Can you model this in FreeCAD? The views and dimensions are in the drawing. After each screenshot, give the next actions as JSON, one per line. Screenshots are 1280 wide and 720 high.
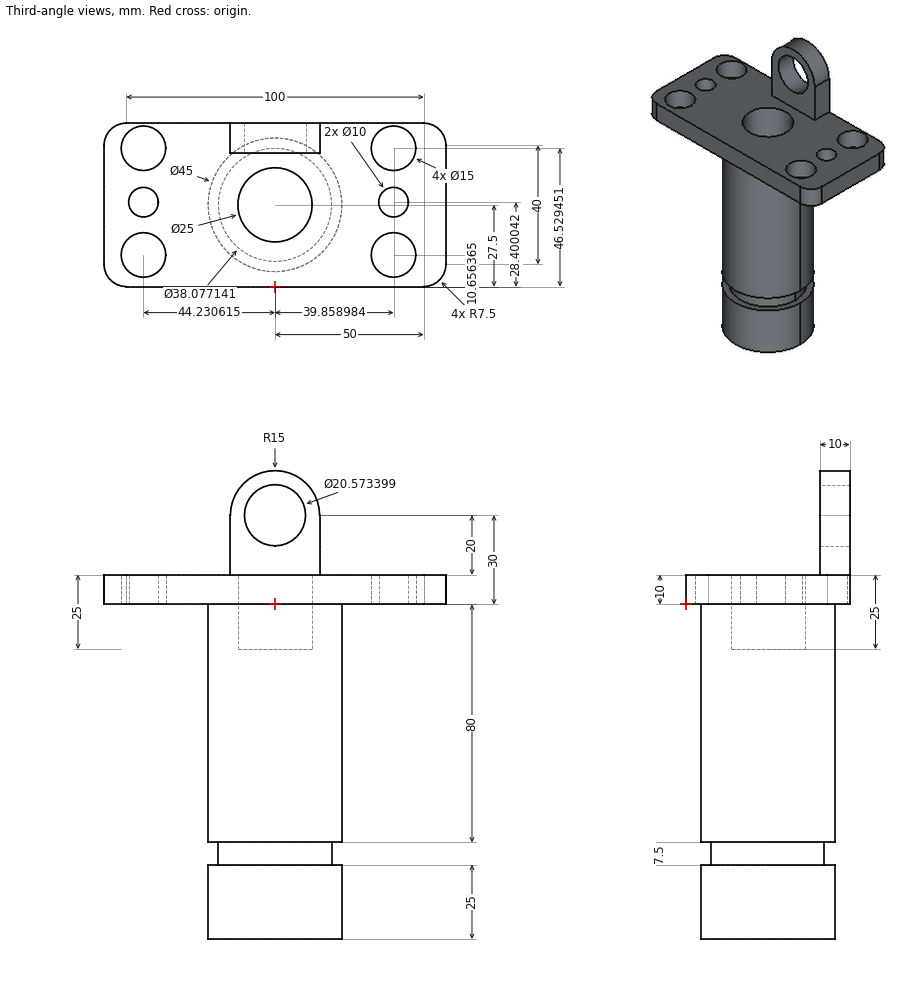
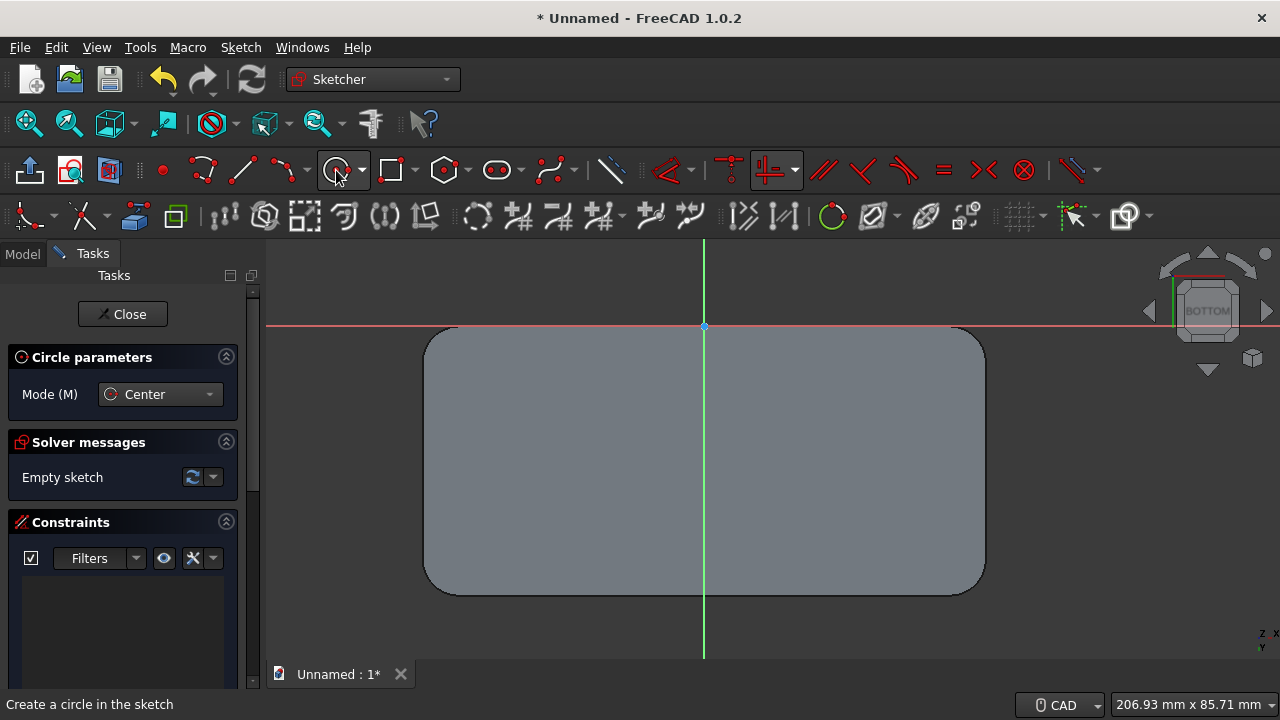
{"action": "left_click", "coordinate": [704, 461]}
{"action": "left_click", "coordinate": [782, 383]}
{"action": "key", "text": "Escape"}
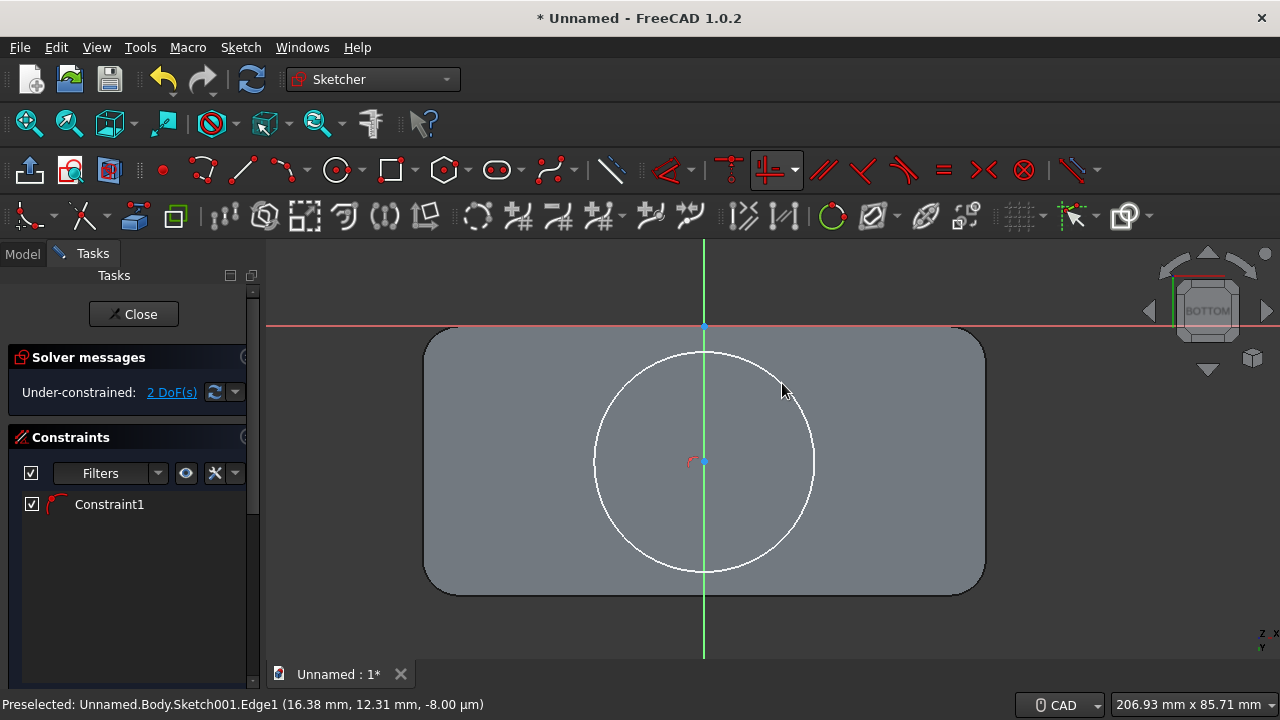
{"action": "left_click", "coordinate": [666, 170]}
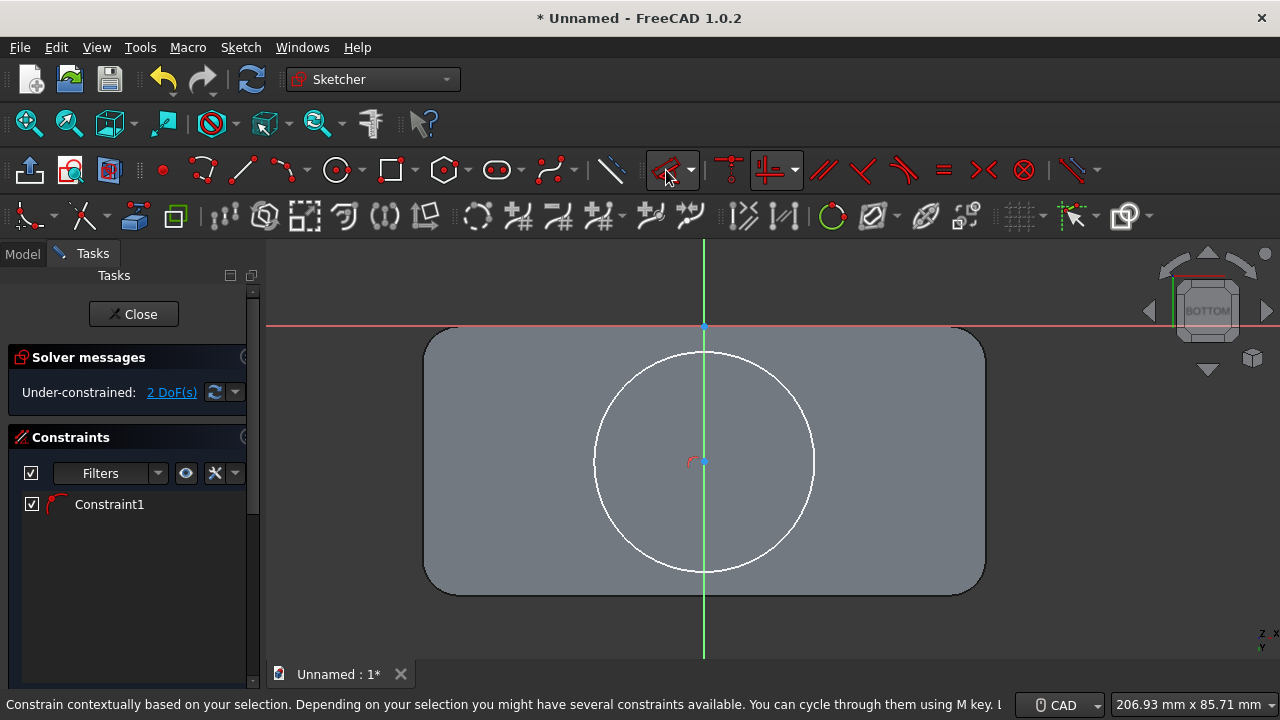
{"action": "left_click", "coordinate": [782, 384]}
{"action": "left_click", "coordinate": [805, 361]}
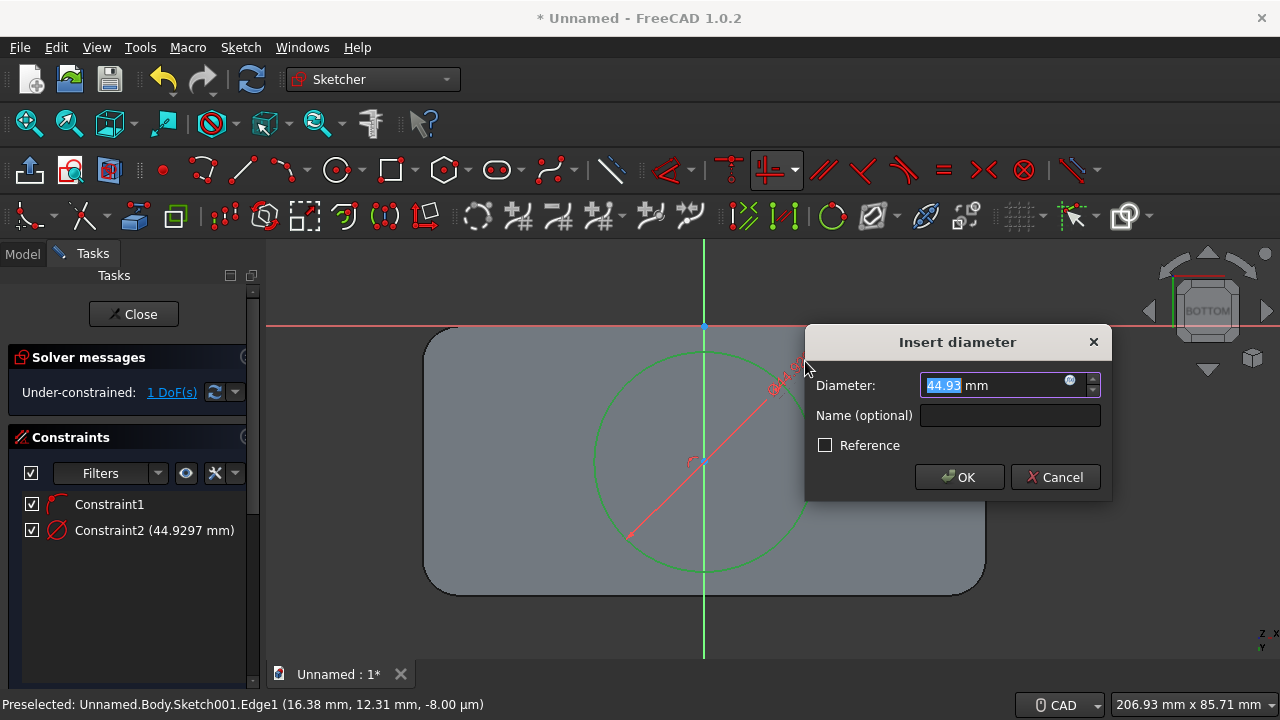
{"action": "type", "text": "45"}
{"action": "key", "text": "Return"}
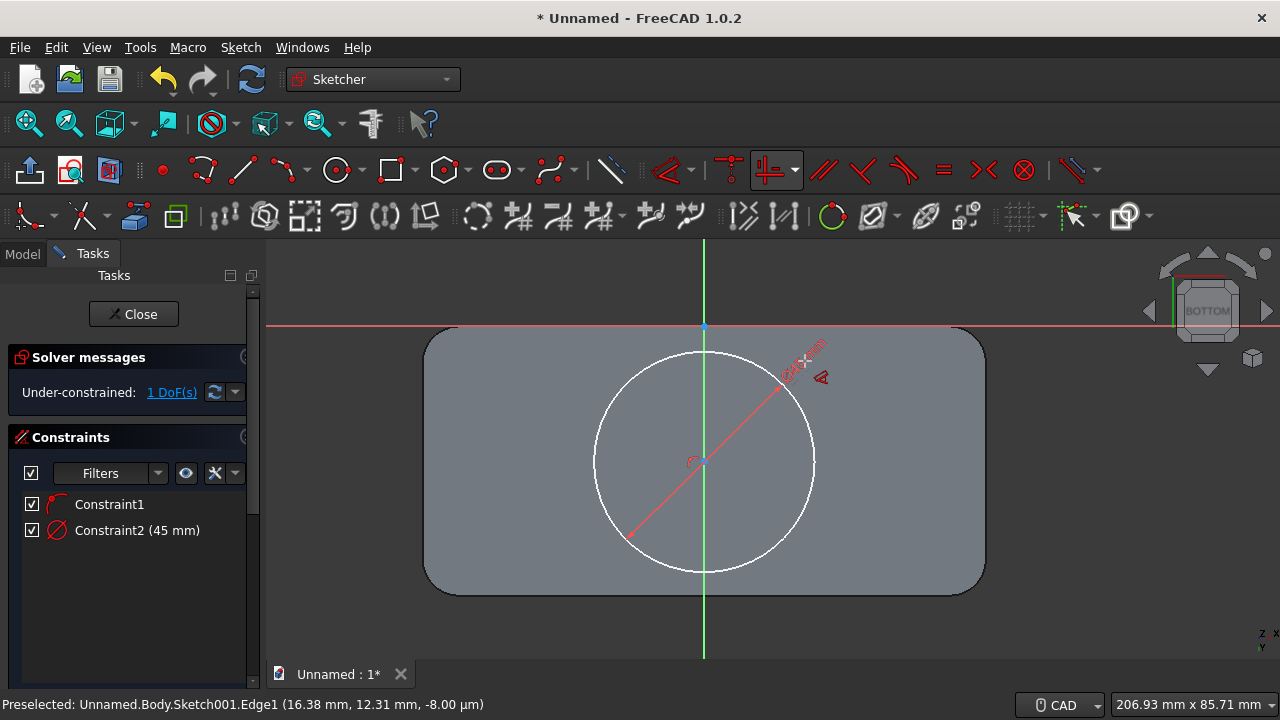
{"action": "left_click", "coordinate": [704, 462]}
{"action": "left_click", "coordinate": [738, 394]}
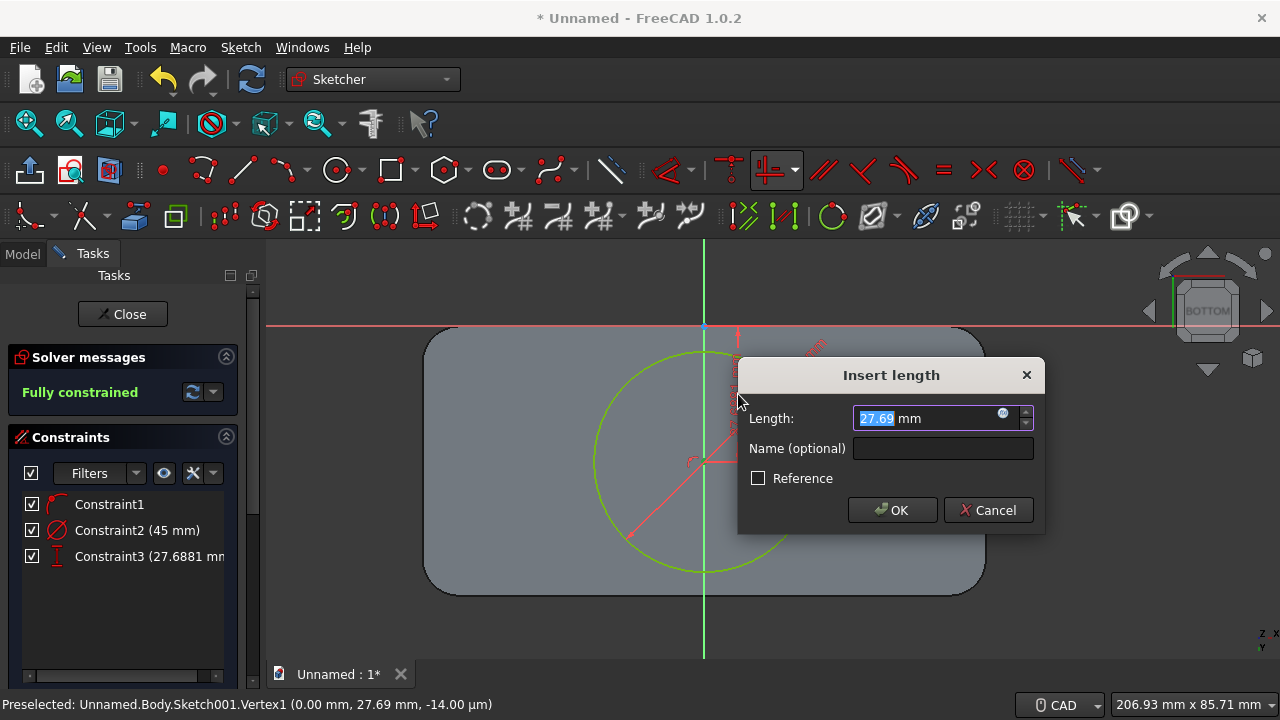
{"action": "type", "text": "27.5"}
{"action": "key", "text": "Return"}
{"action": "key", "text": "Escape"}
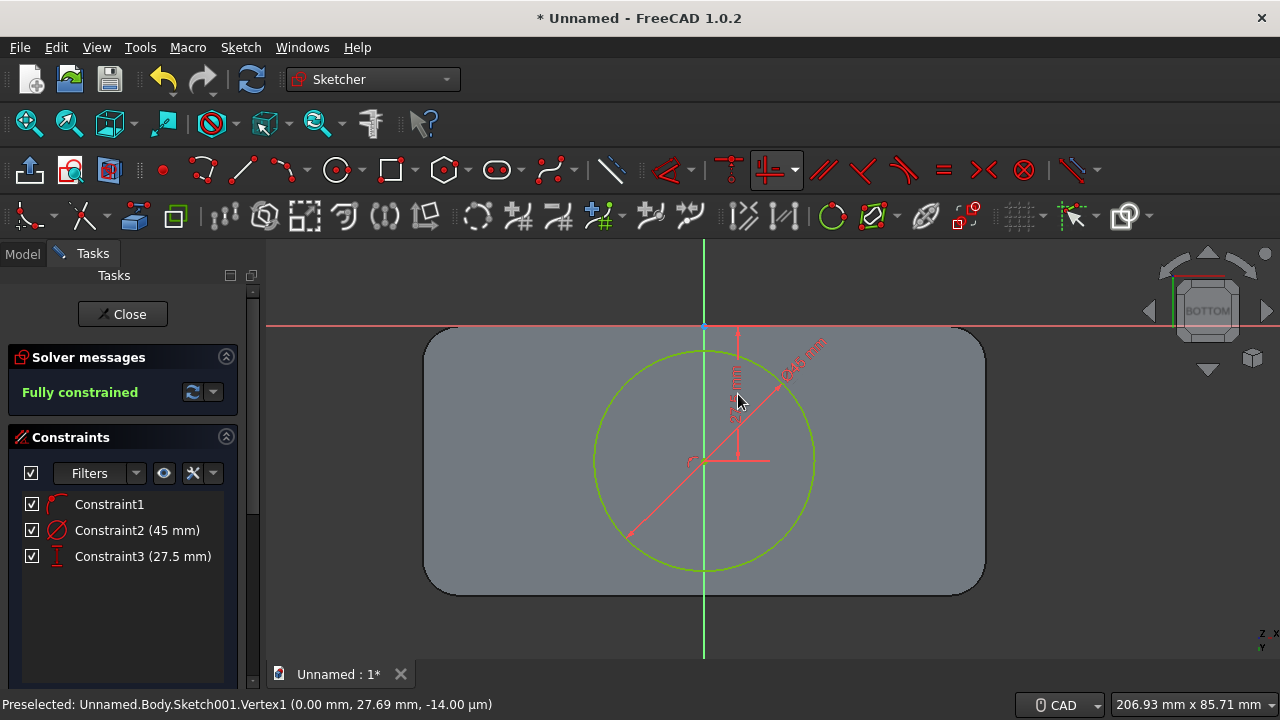
{"action": "left_click", "coordinate": [123, 314]}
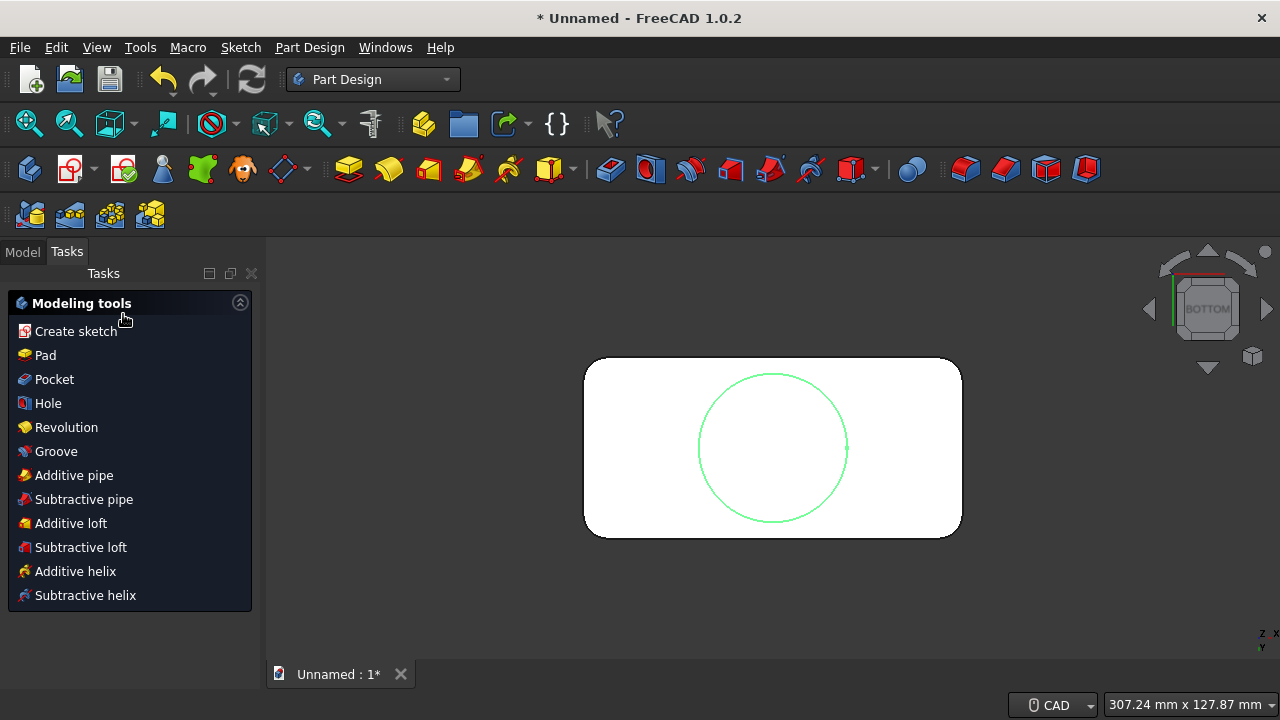
{"action": "left_click", "coordinate": [350, 170]}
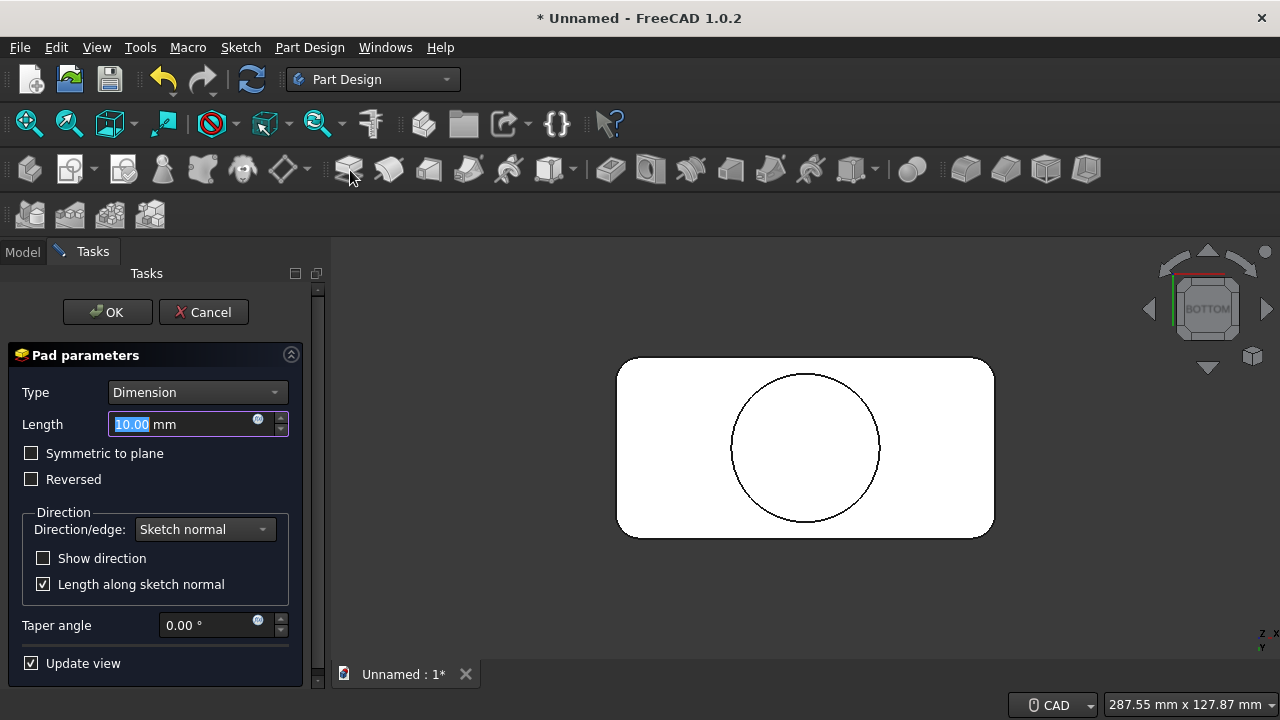
{"action": "type", "text": "80"}
{"action": "key", "text": "Tab"}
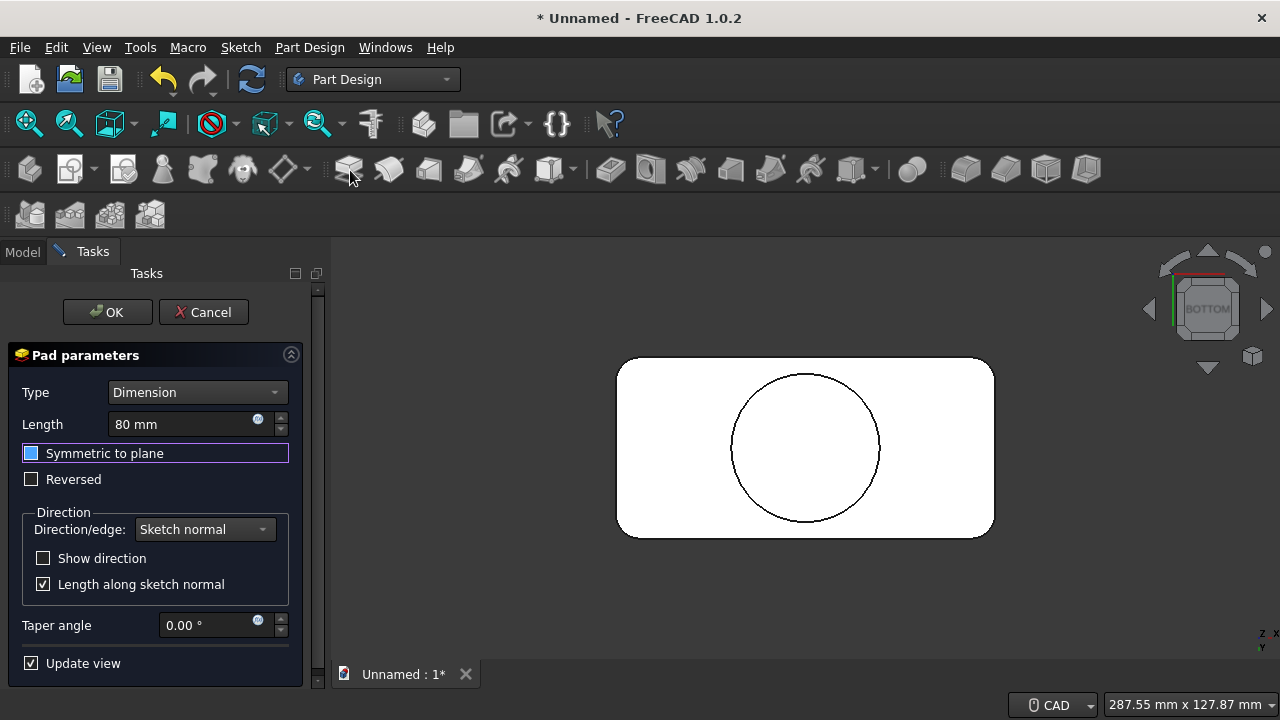
{"action": "left_click", "coordinate": [108, 312]}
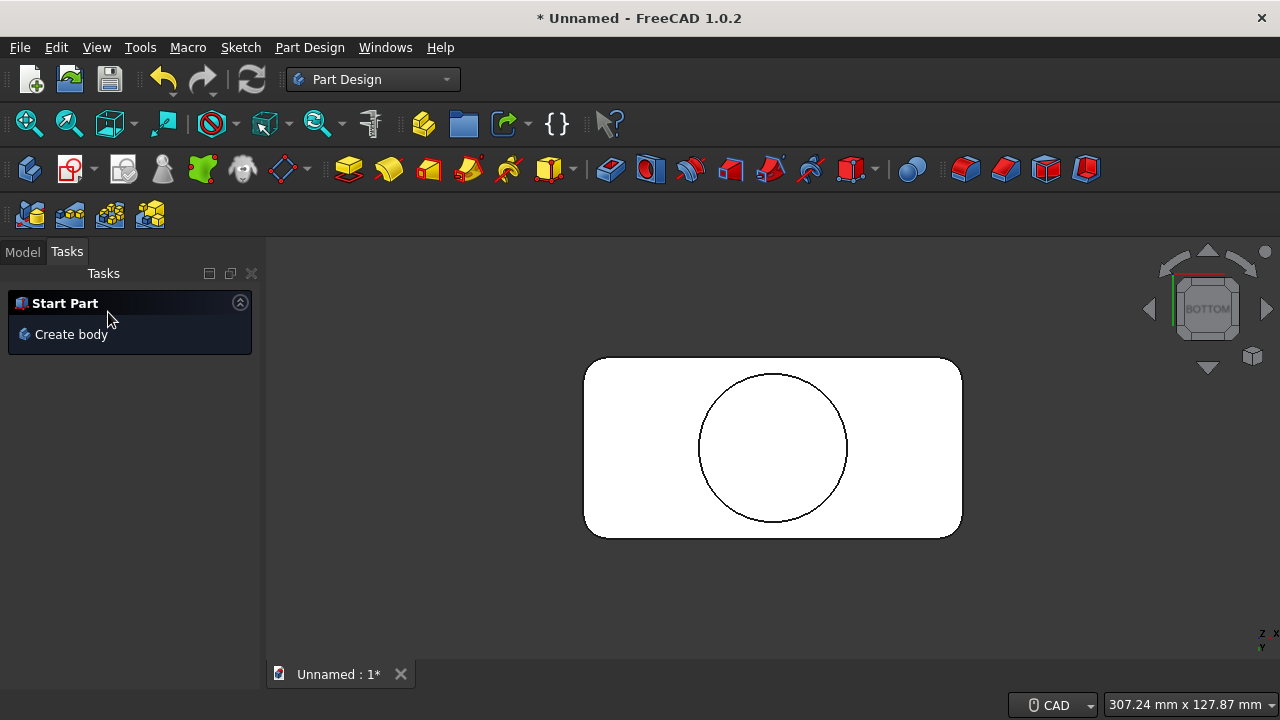
{"action": "left_click", "coordinate": [30, 124]}